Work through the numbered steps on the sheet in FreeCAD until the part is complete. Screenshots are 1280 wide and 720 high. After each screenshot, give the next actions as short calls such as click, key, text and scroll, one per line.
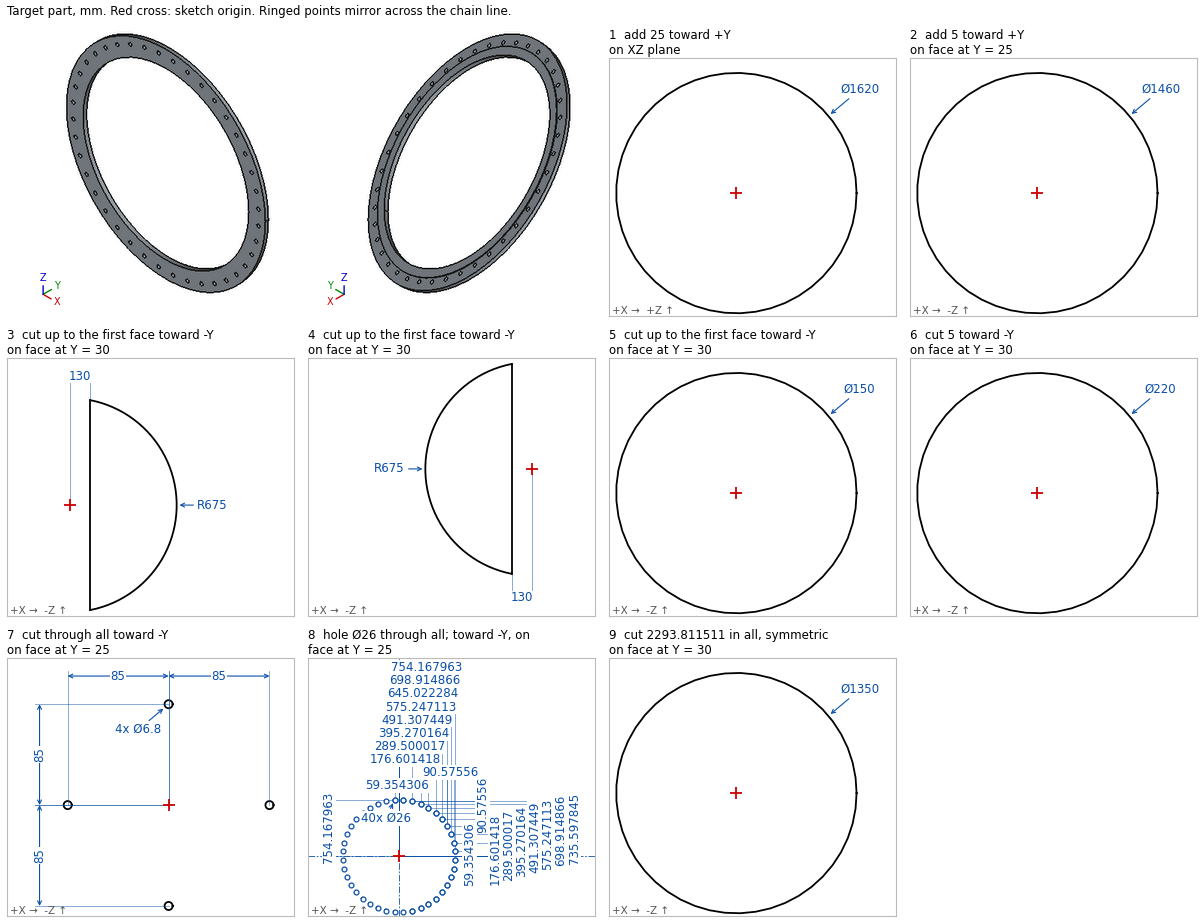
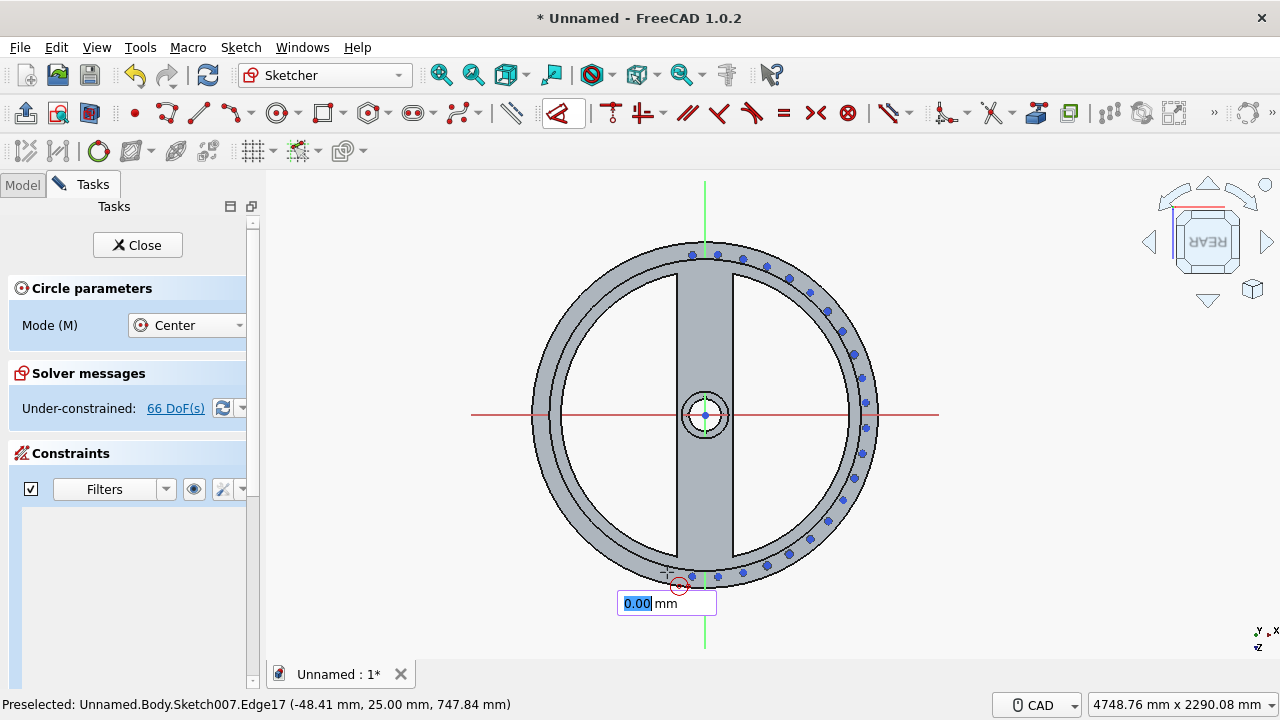
scroll(669, 570, up, 9)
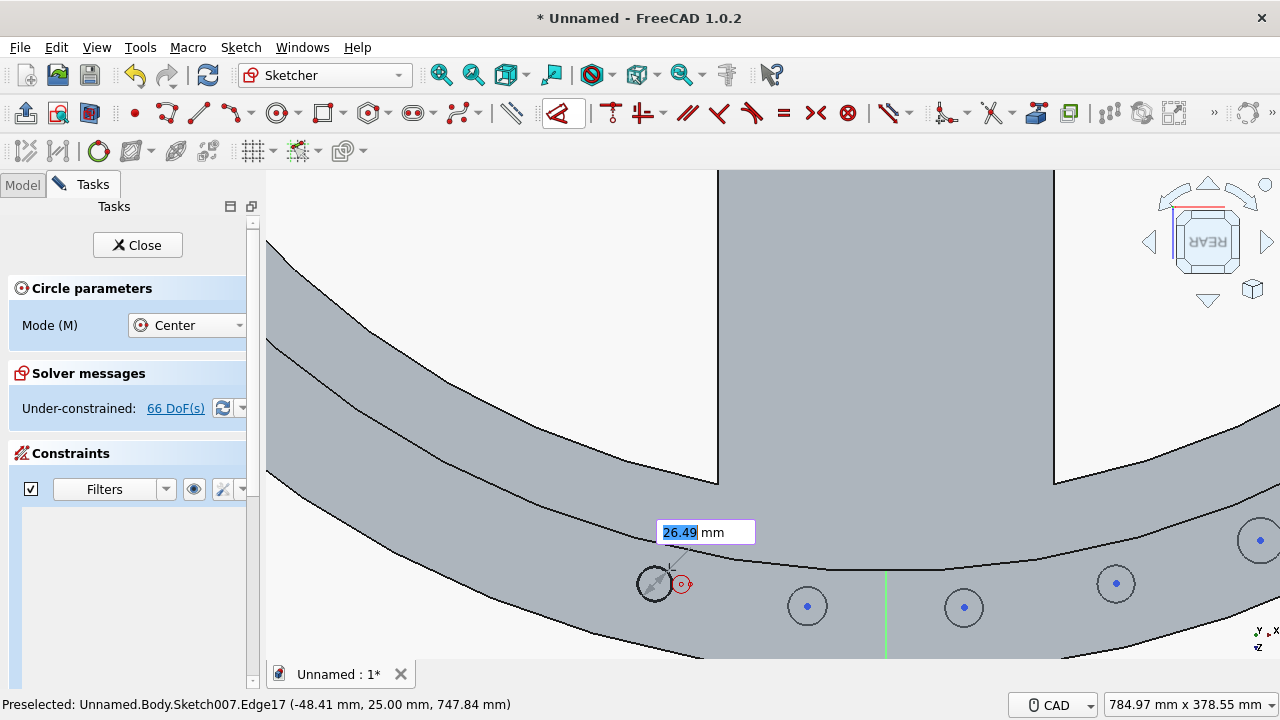
click(669, 567)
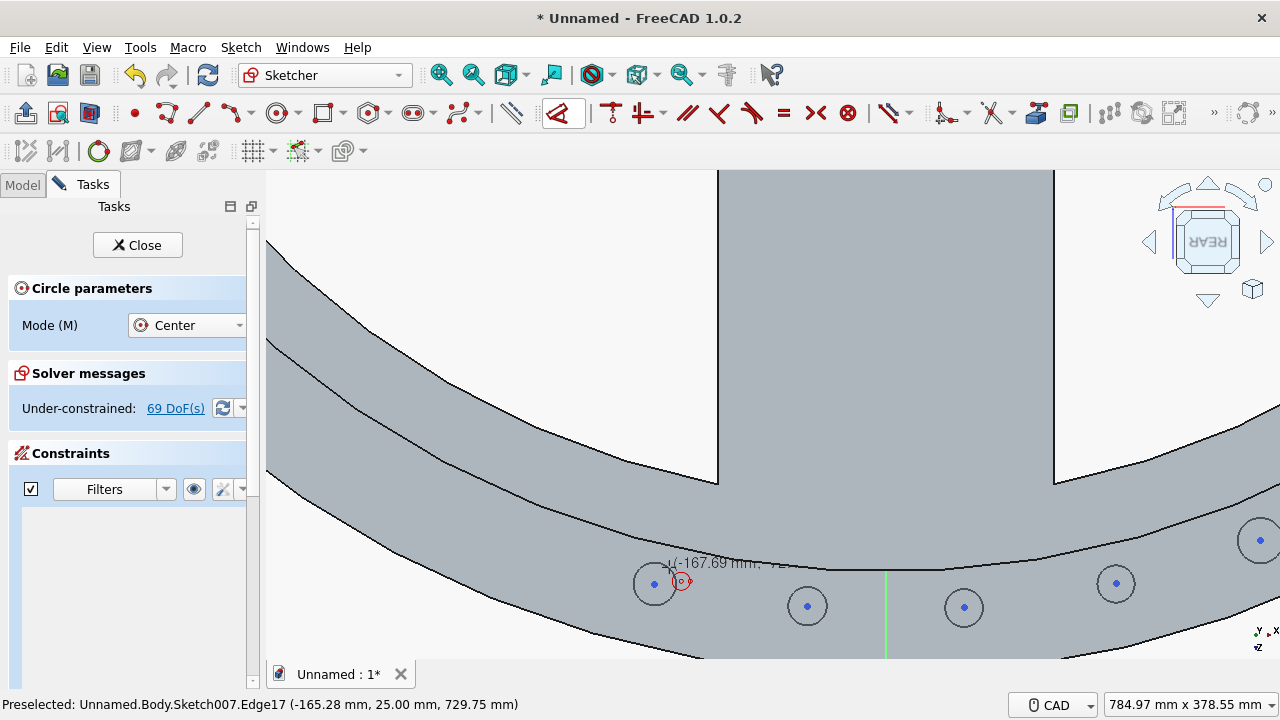
scroll(512, 532, up, 2)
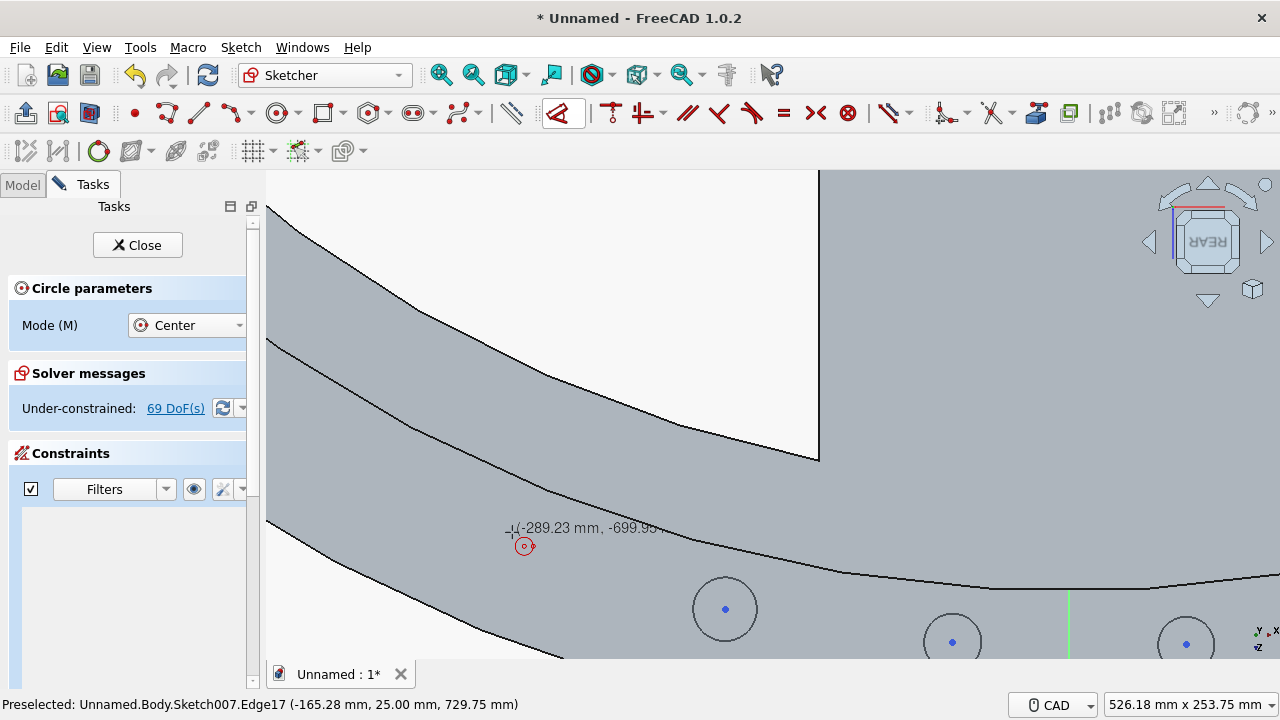
scroll(659, 568, down, 11)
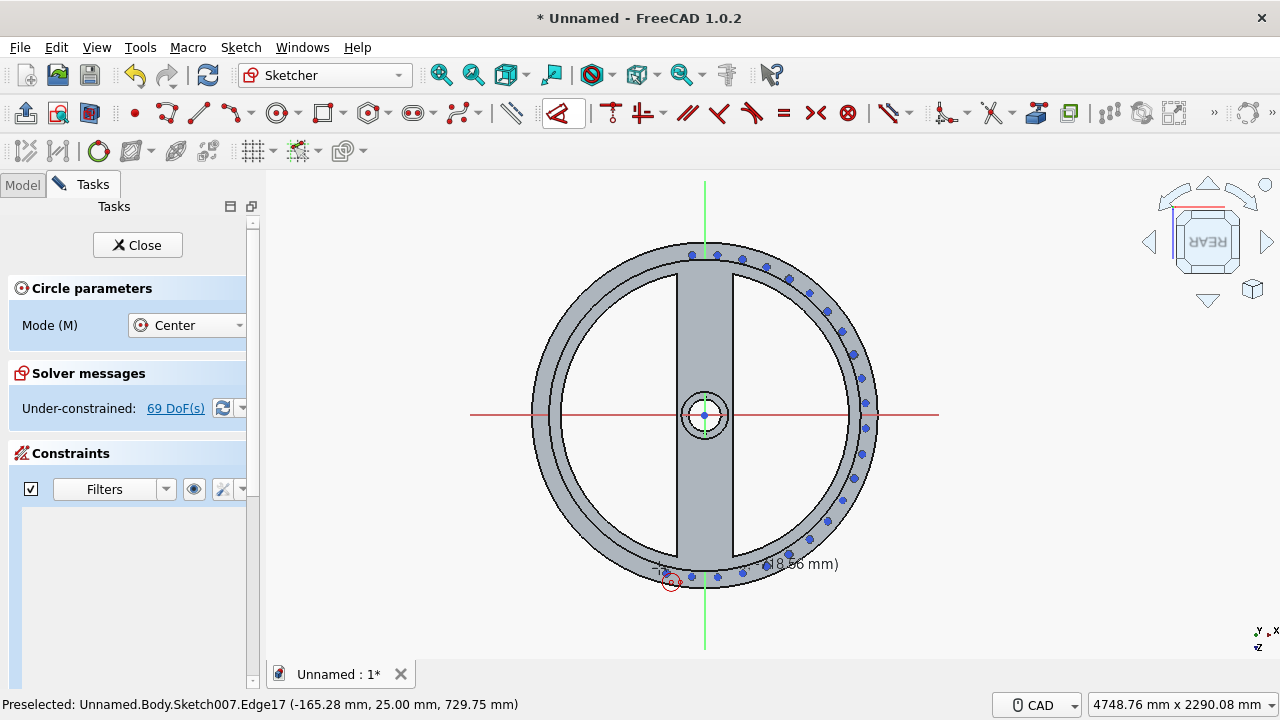
click(643, 565)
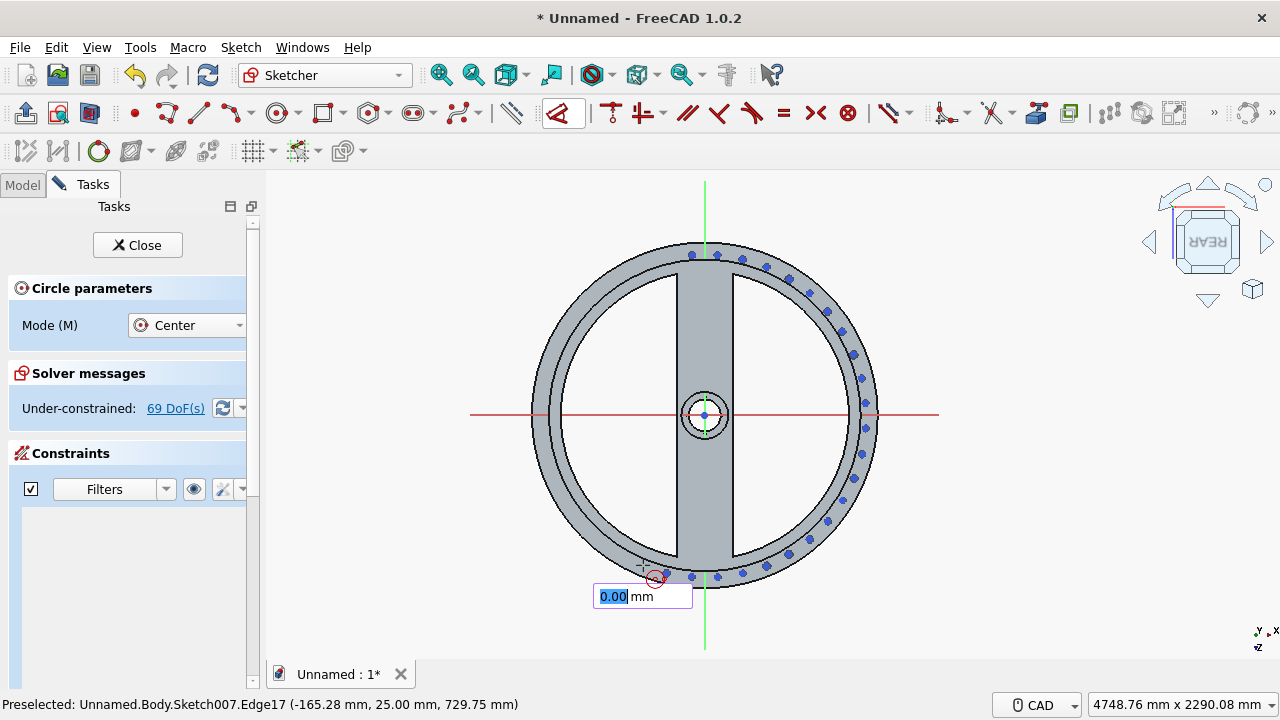
scroll(645, 563, up, 9)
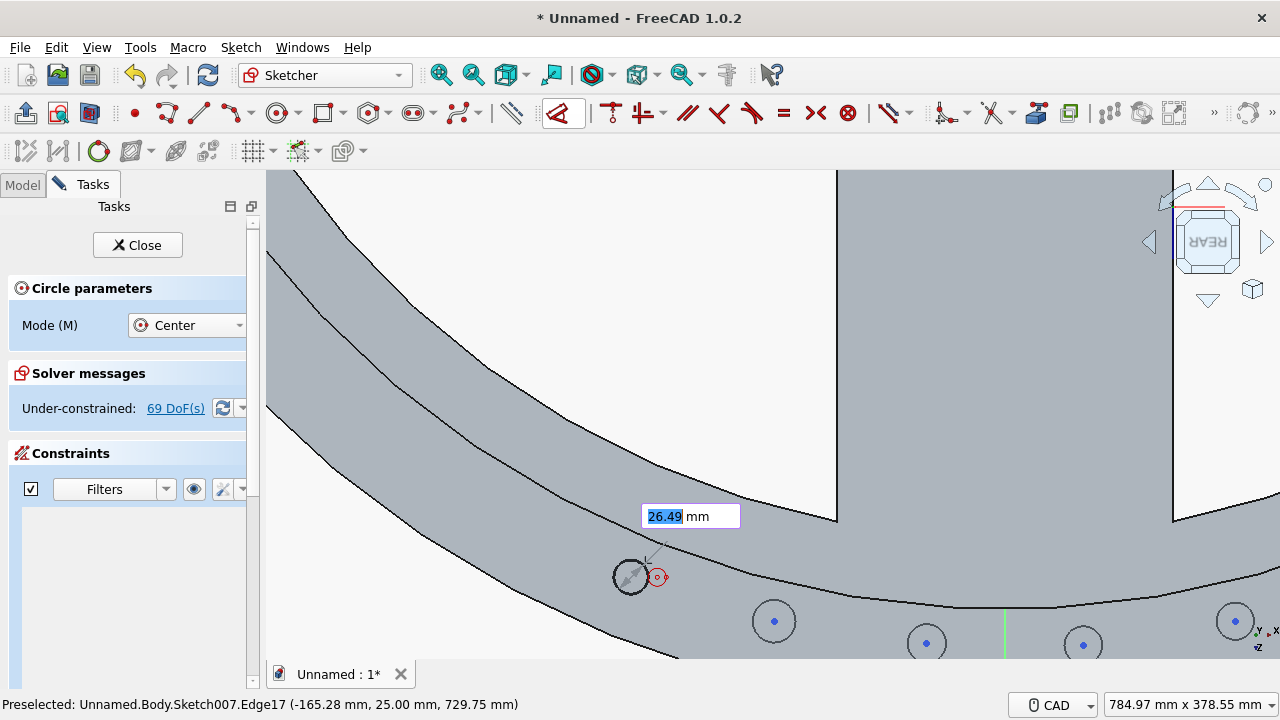
click(643, 557)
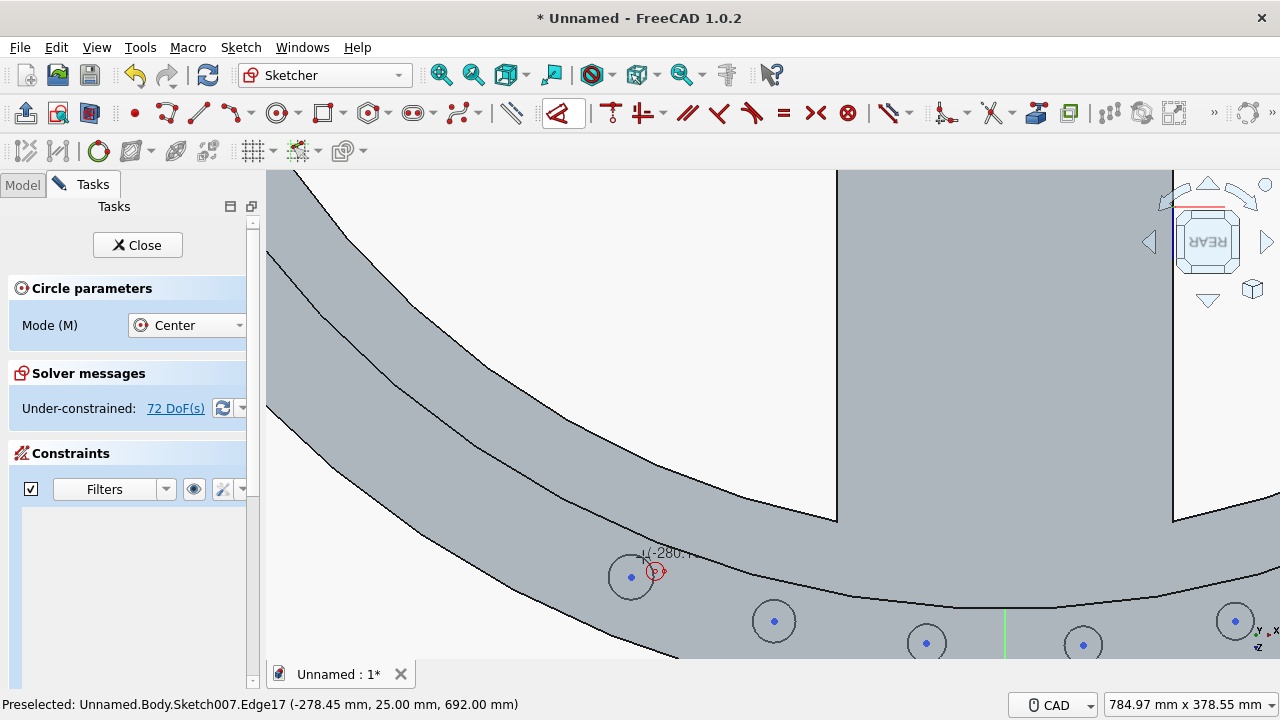
scroll(494, 499, up, 2)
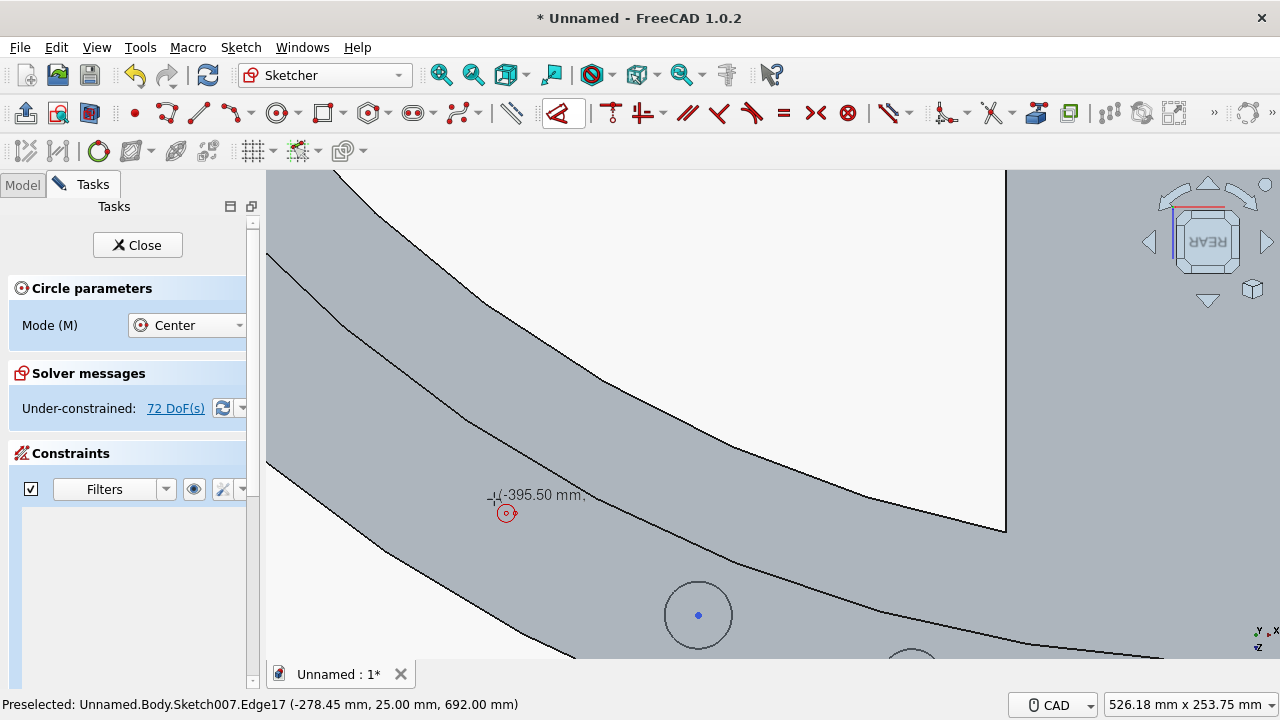
scroll(636, 559, down, 11)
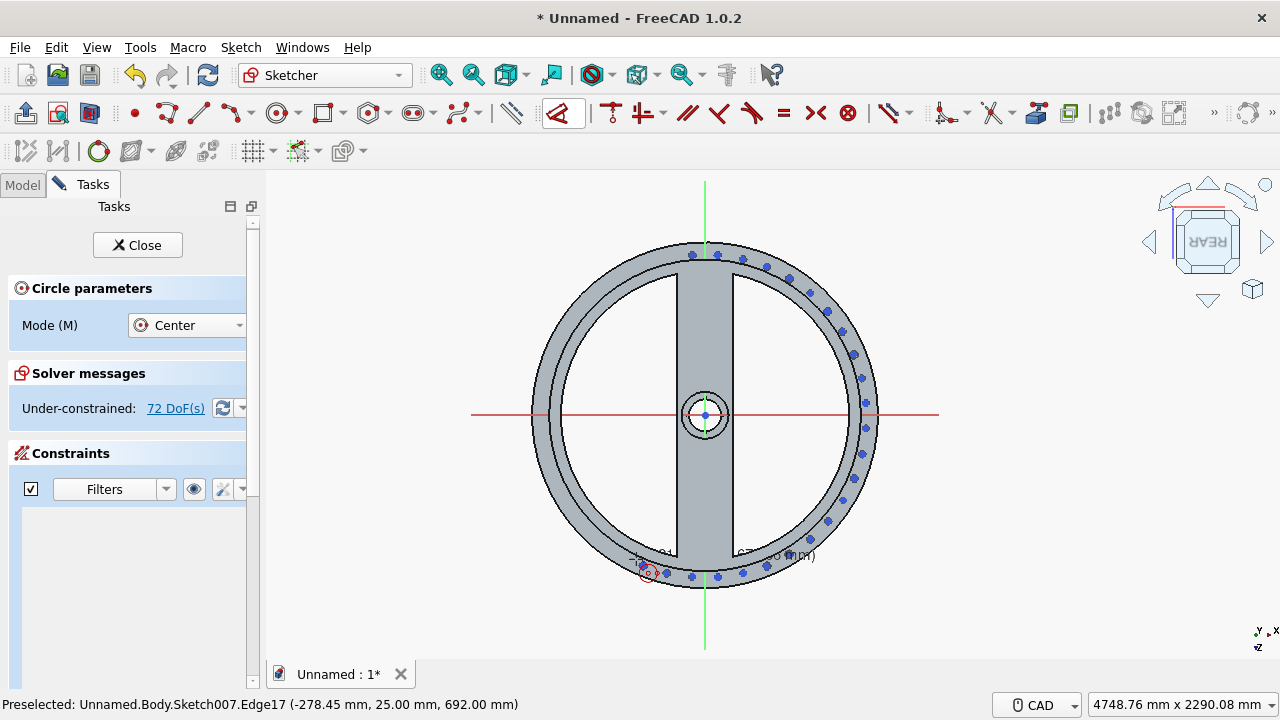
click(621, 553)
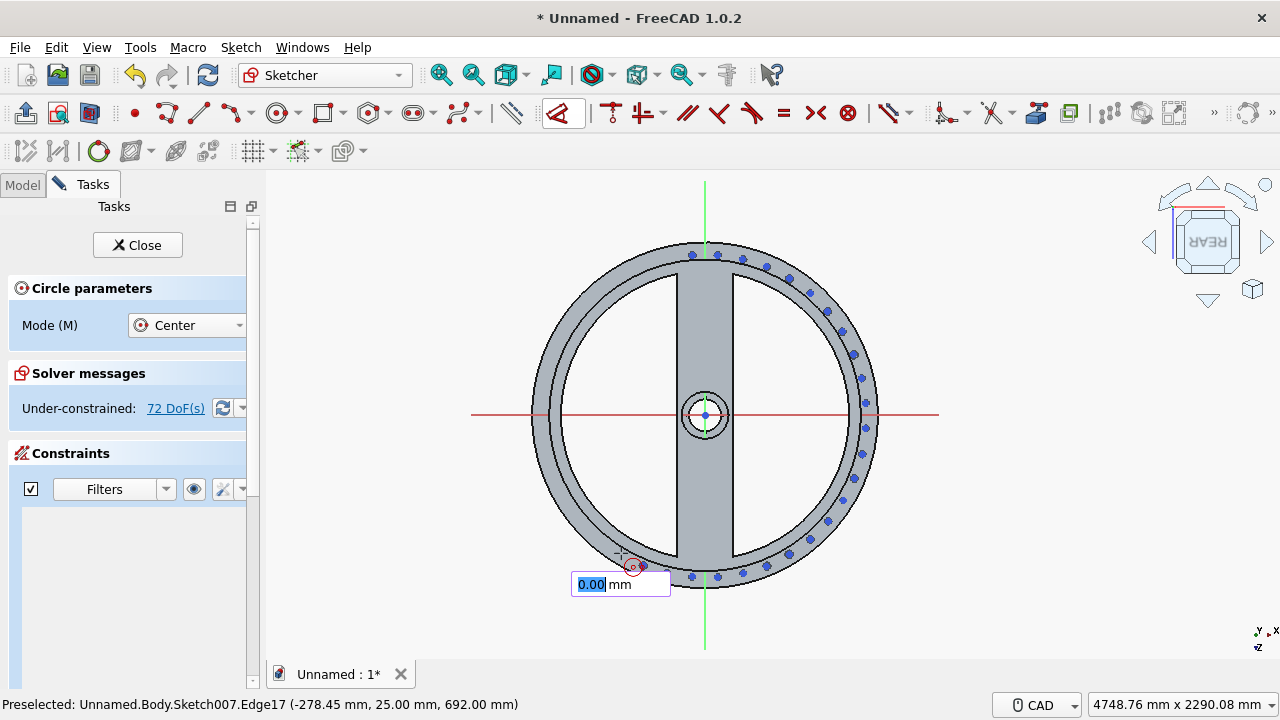
scroll(623, 551, up, 9)